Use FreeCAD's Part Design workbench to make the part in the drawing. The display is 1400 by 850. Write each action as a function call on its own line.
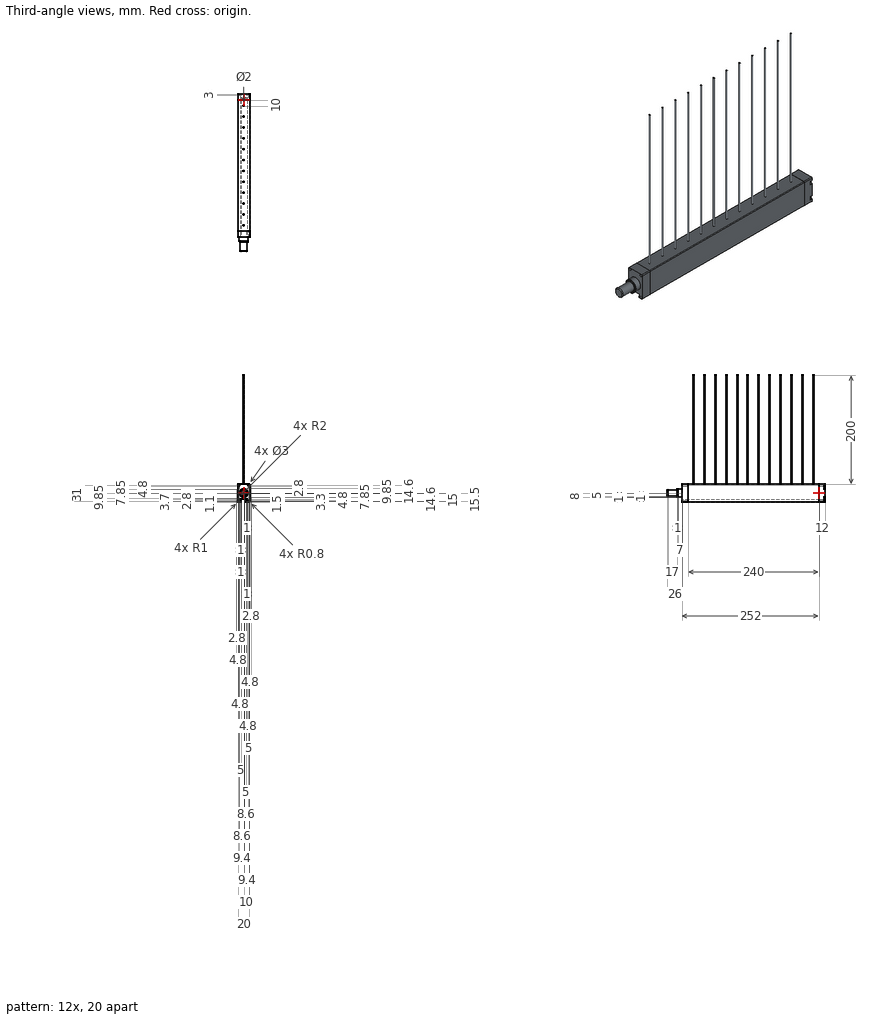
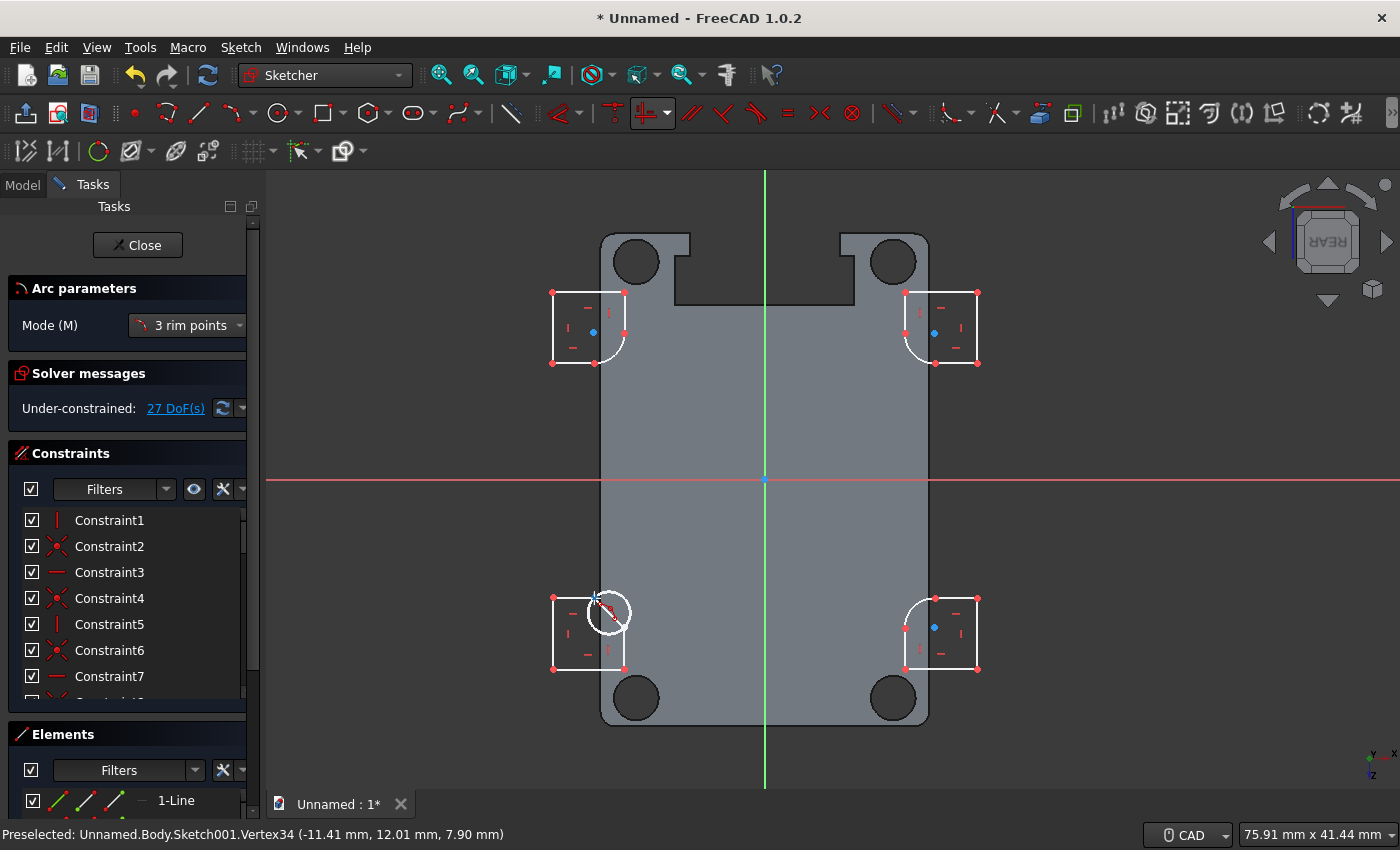
scroll(616, 606, up, 3)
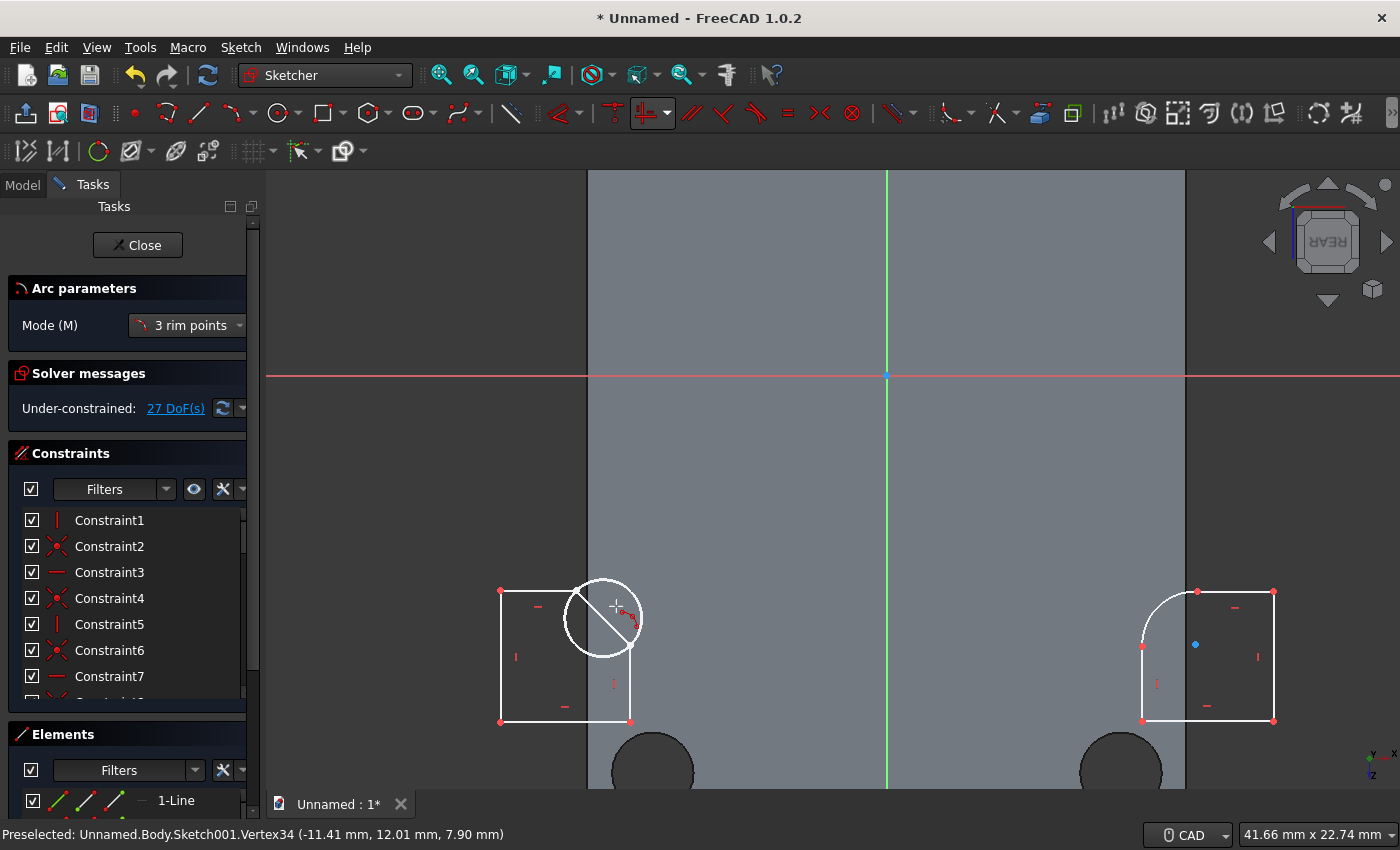
click(615, 605)
key(Escape)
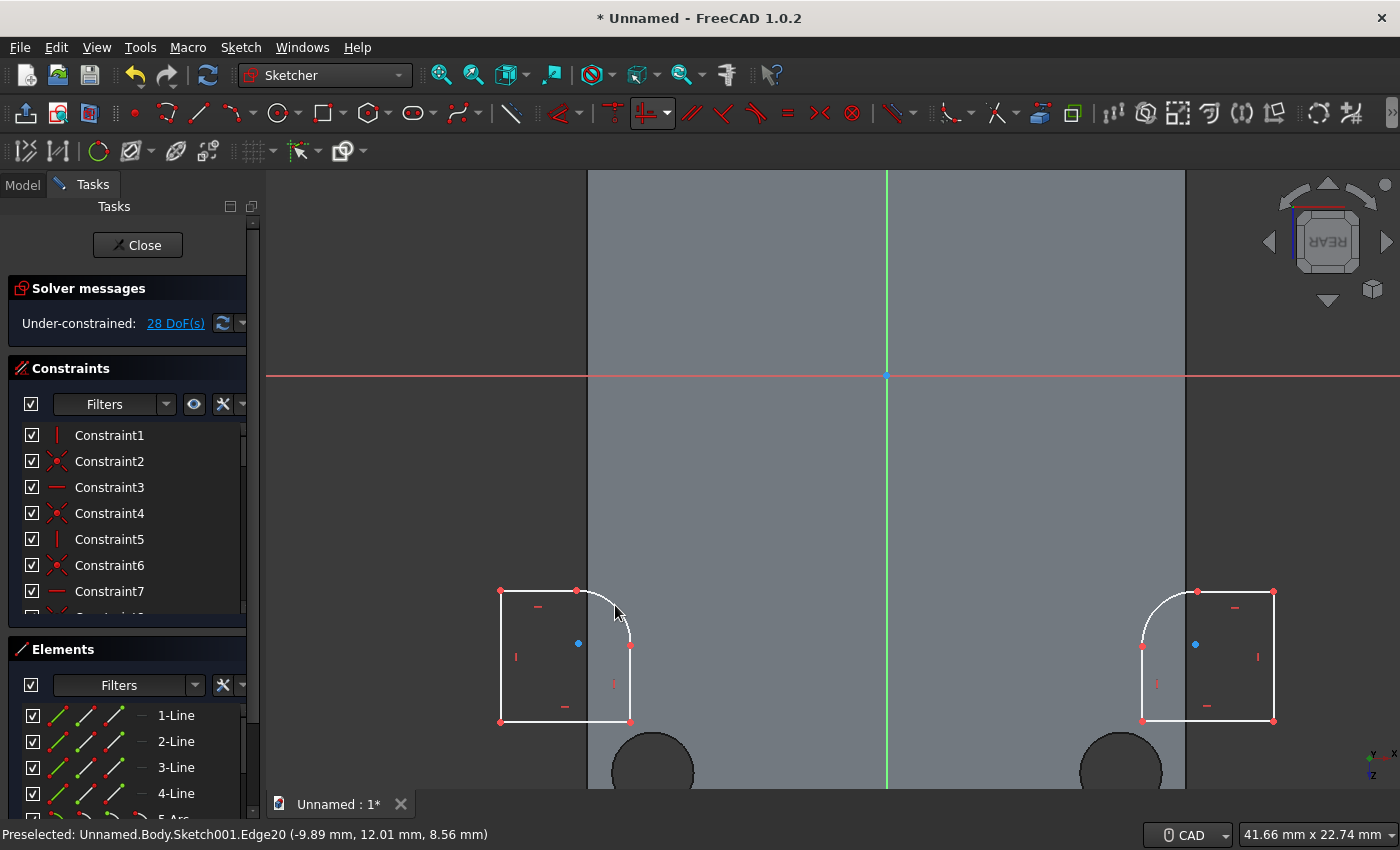
scroll(616, 606, down, 3)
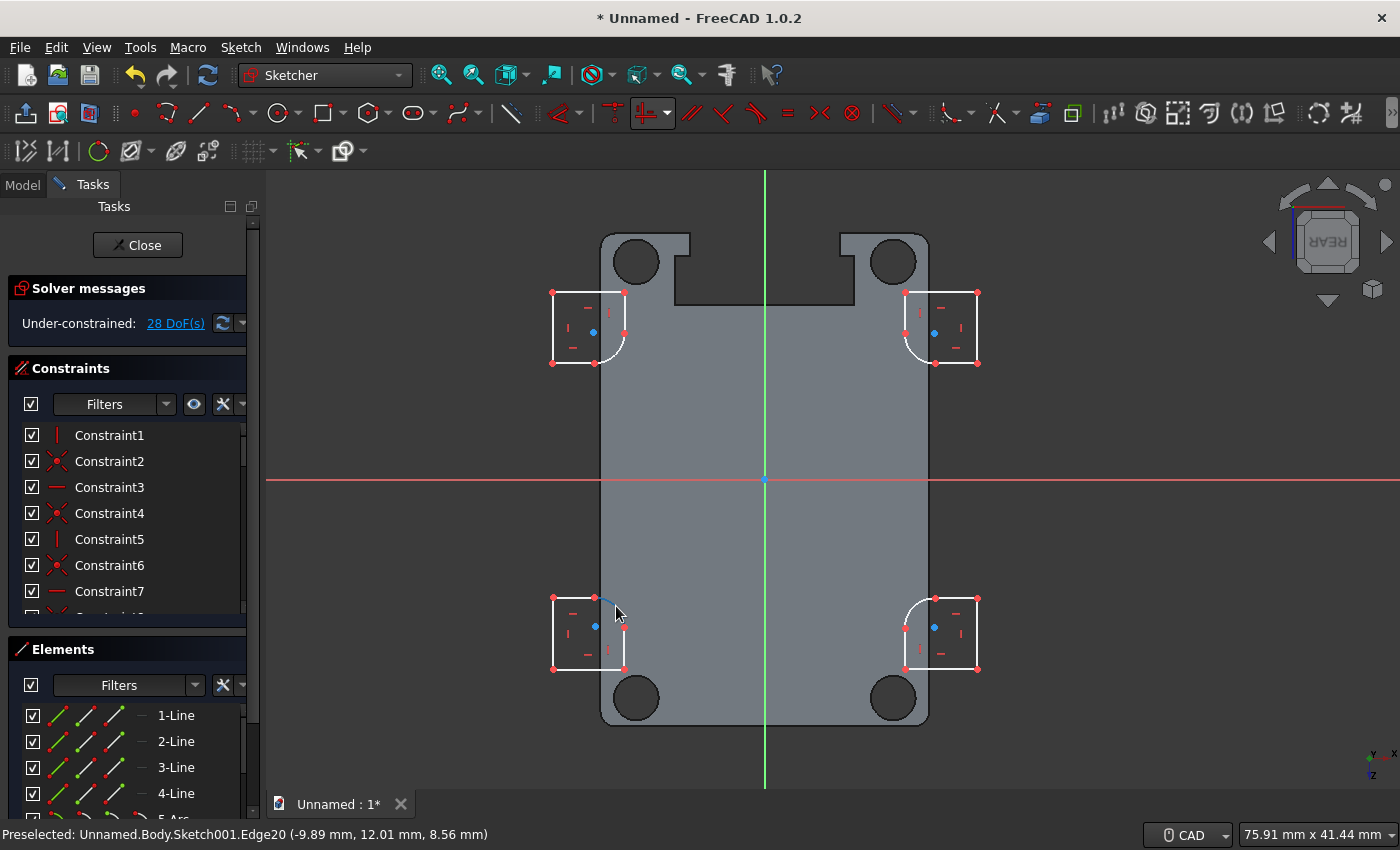
click(625, 321)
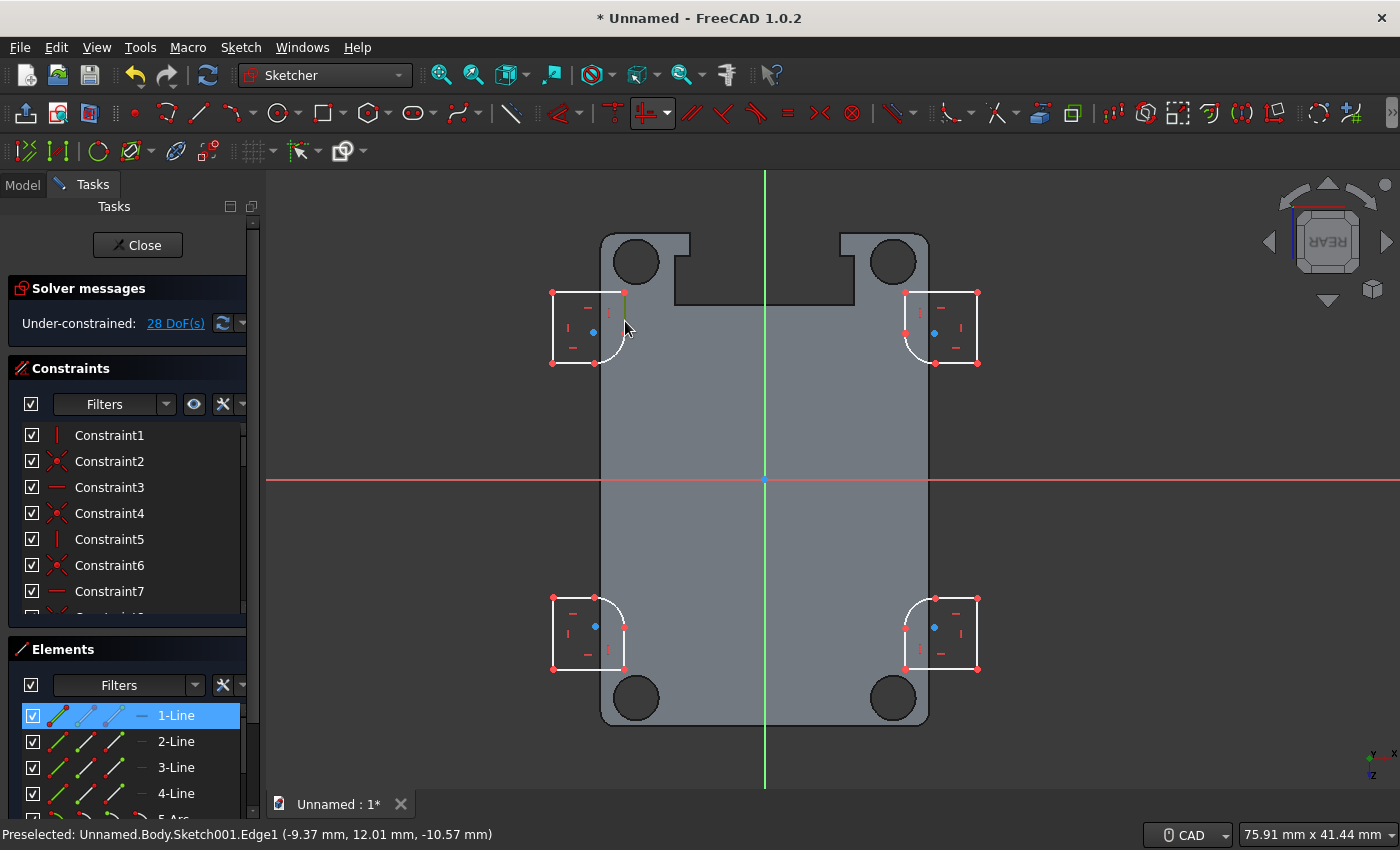
click(608, 360)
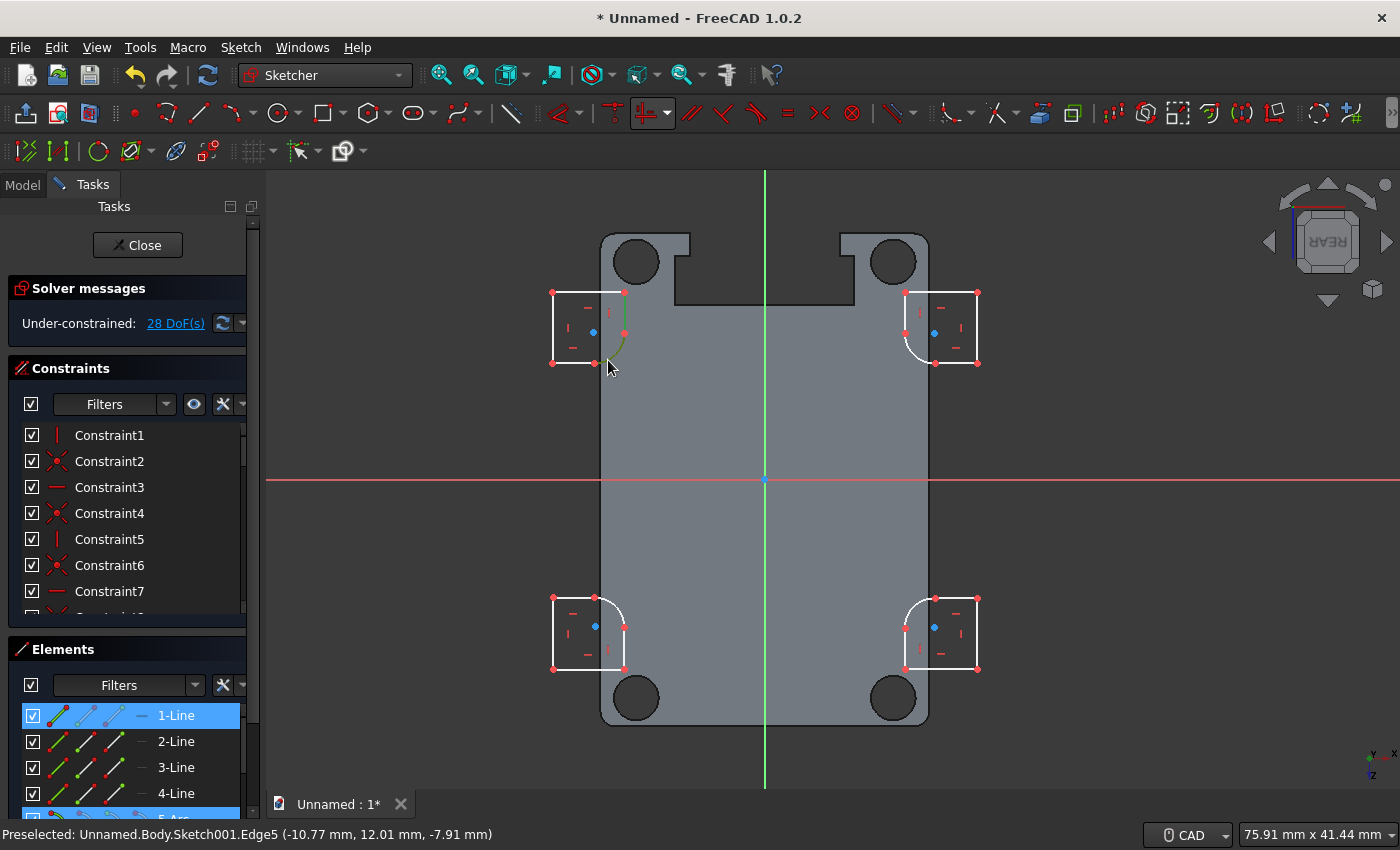
click(756, 114)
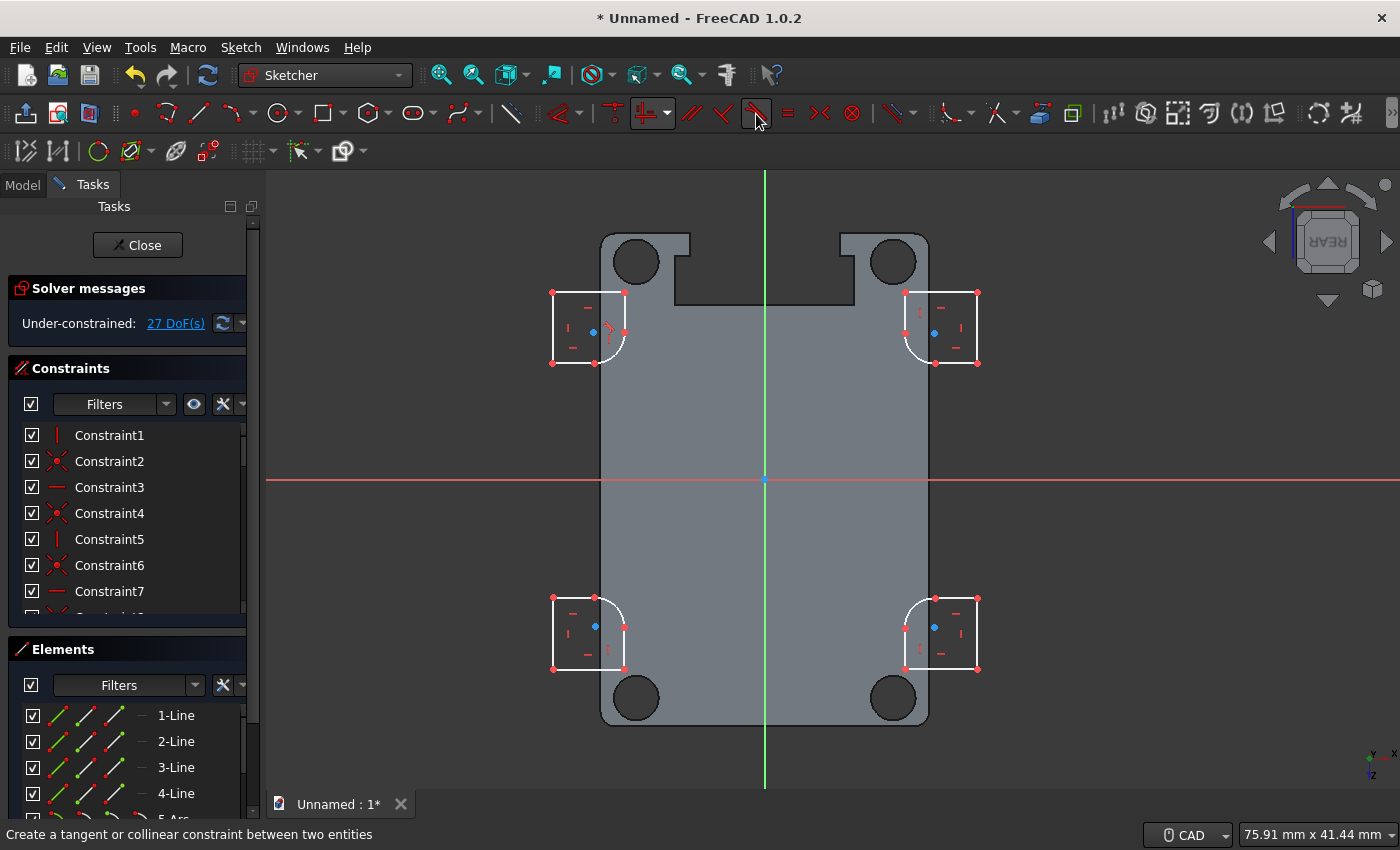
click(565, 363)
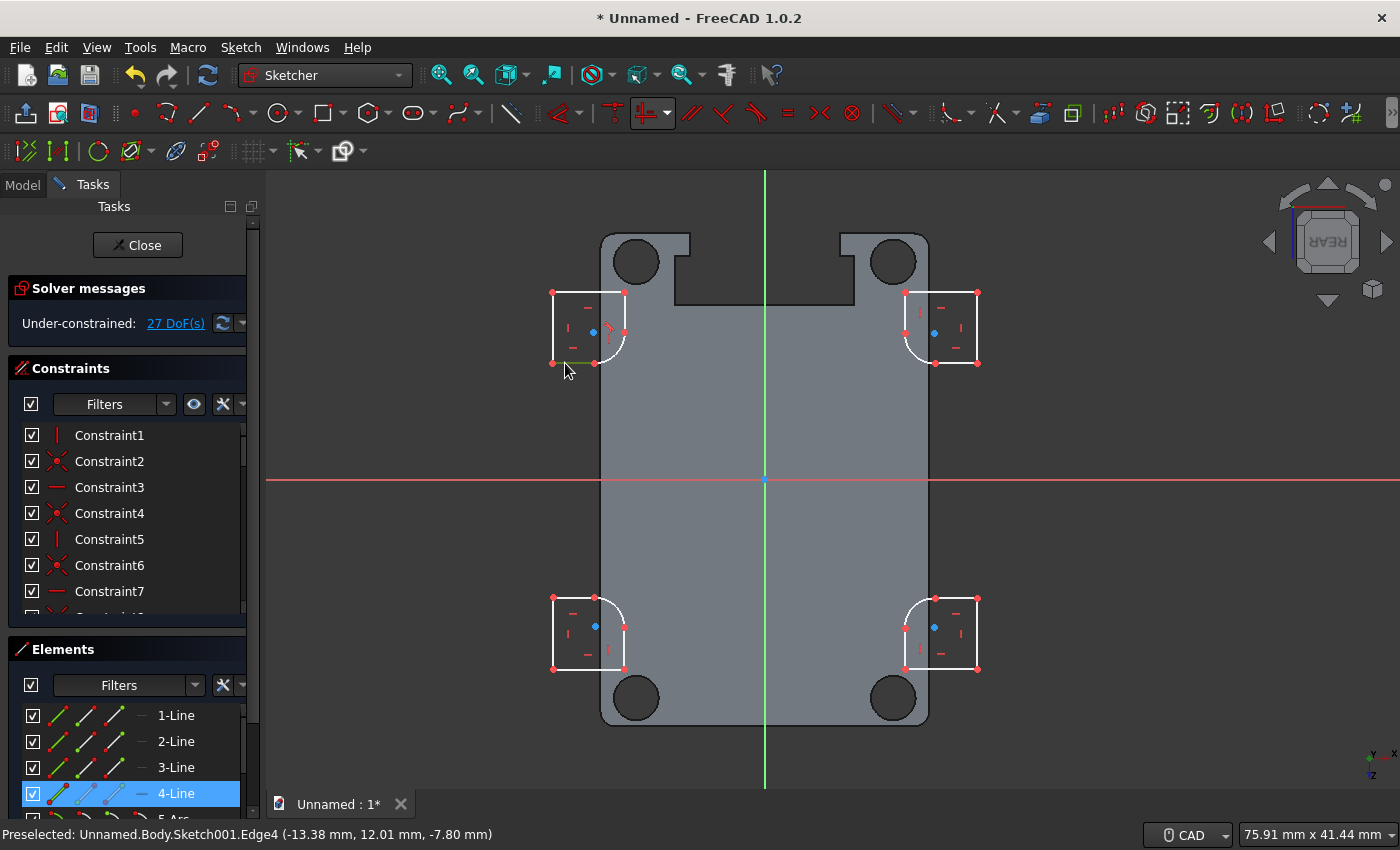
click(608, 360)